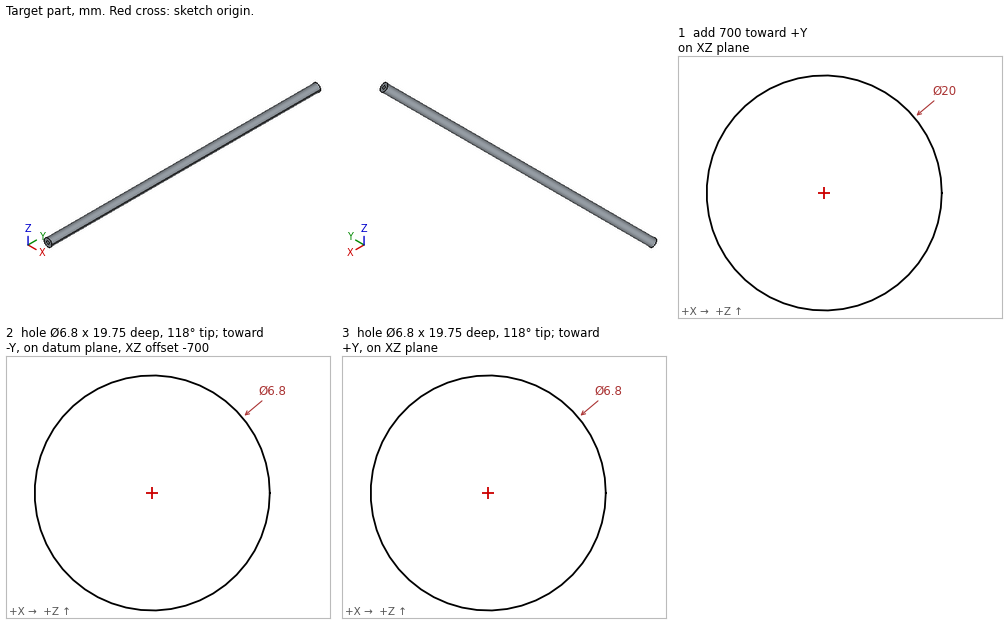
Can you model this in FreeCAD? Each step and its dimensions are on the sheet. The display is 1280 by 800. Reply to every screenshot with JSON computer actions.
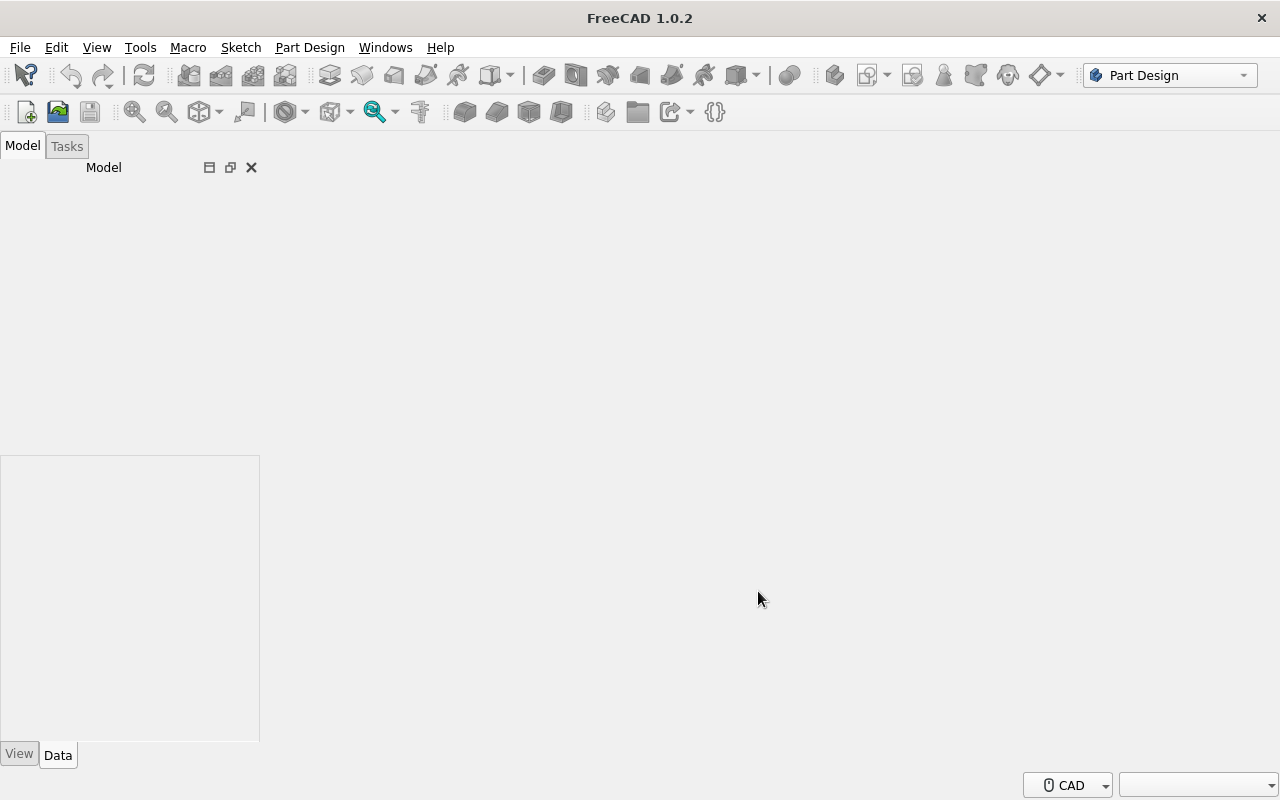
{"action": "left_click", "coordinate": [26, 112]}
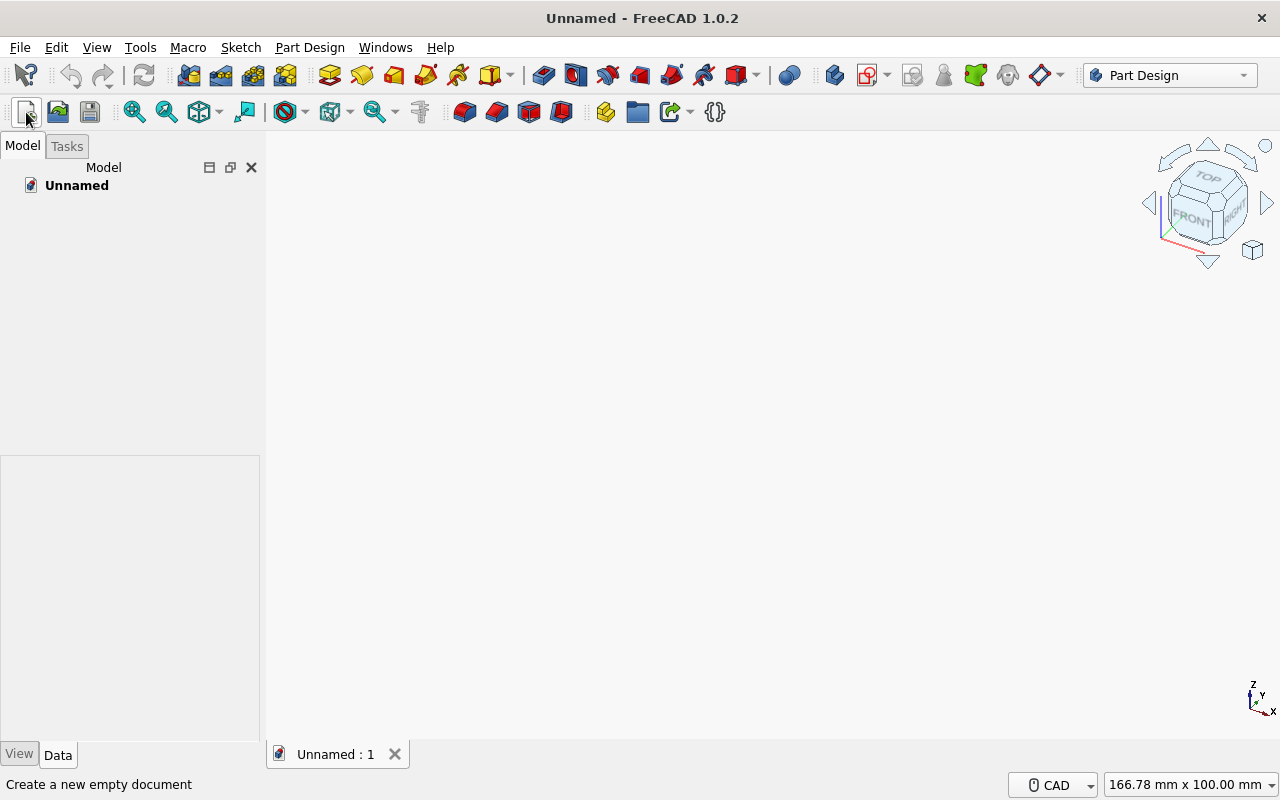
{"action": "left_click", "coordinate": [868, 76]}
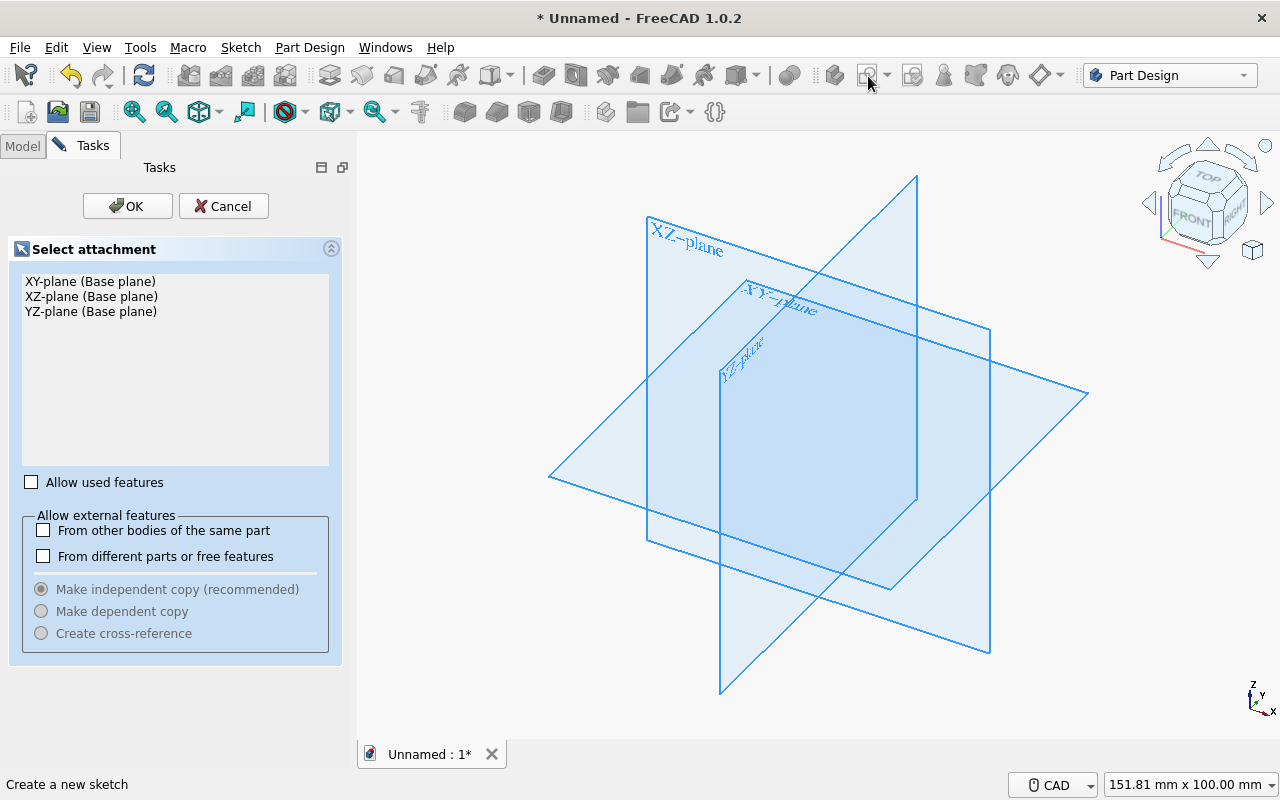
{"action": "left_click", "coordinate": [82, 296]}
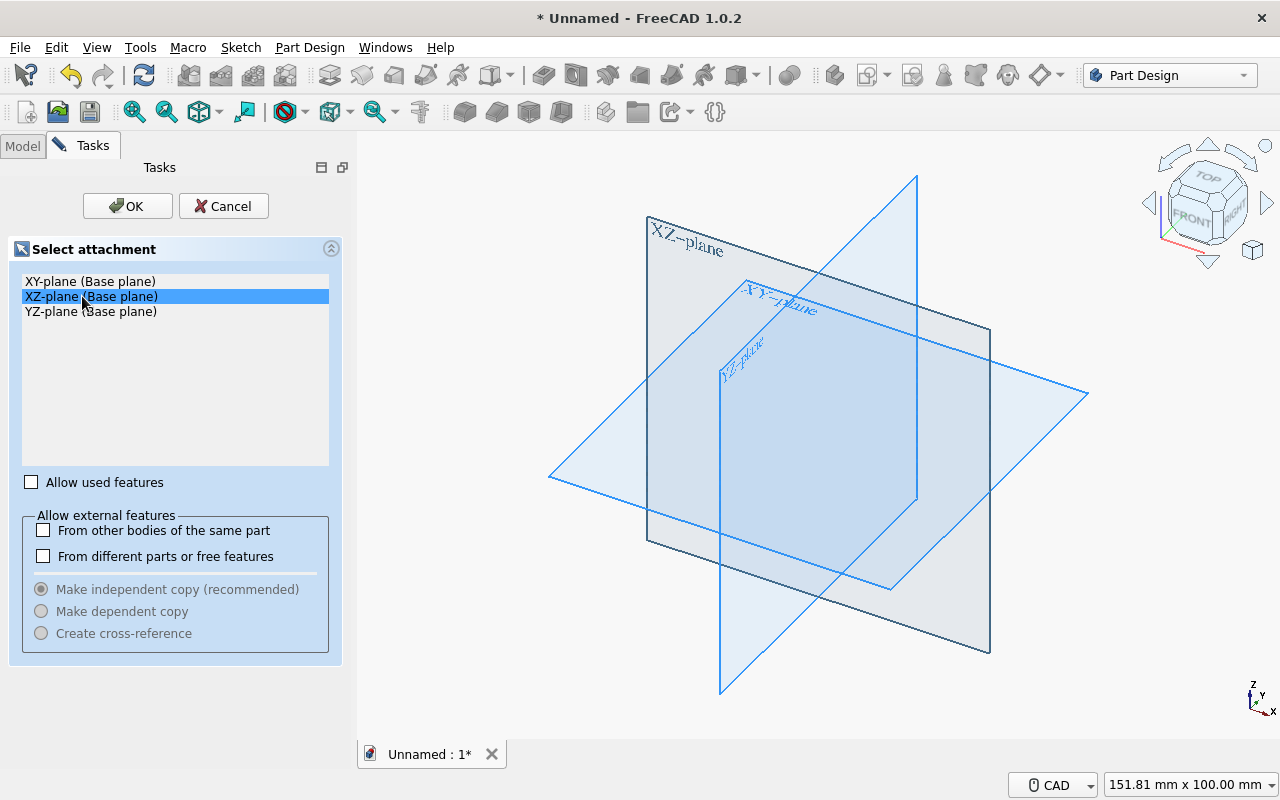
{"action": "left_click", "coordinate": [128, 206]}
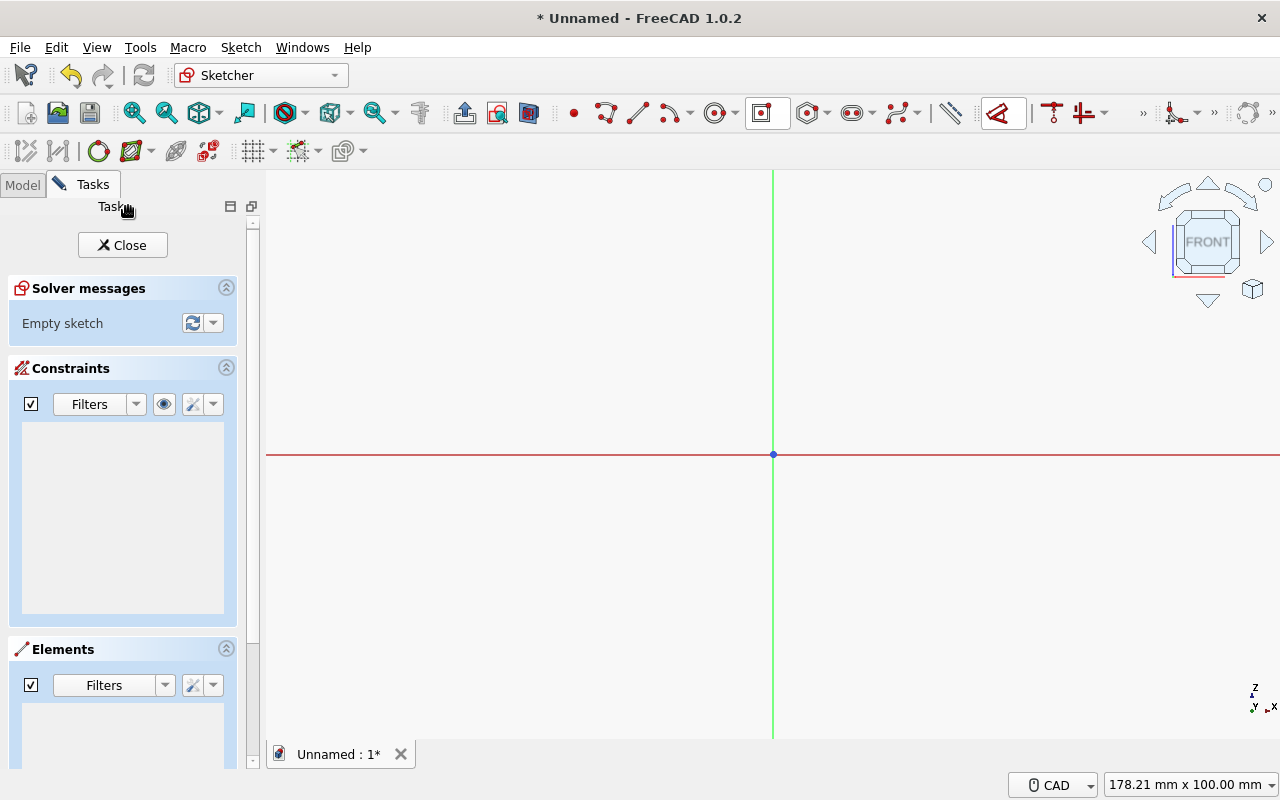
{"action": "scroll", "coordinate": [803, 455], "scroll_direction": "up", "scroll_amount": 6}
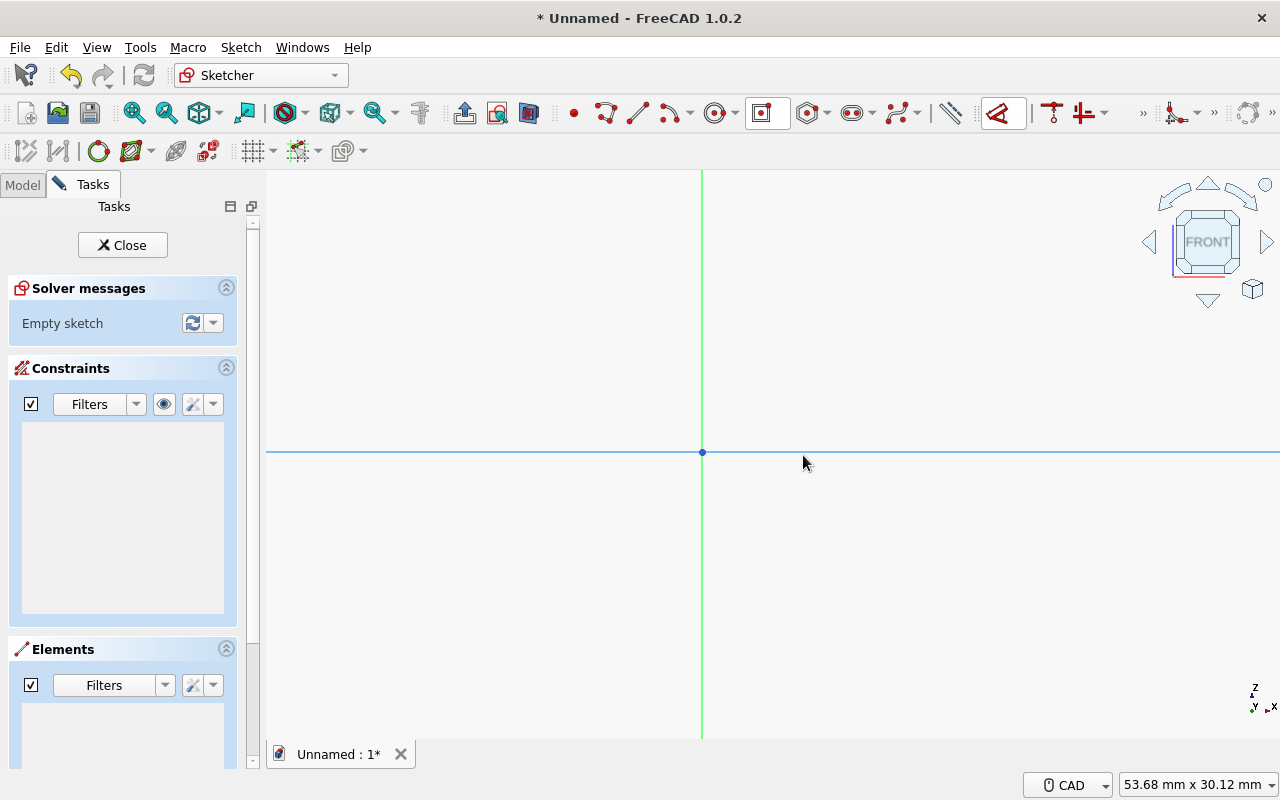
{"action": "left_click", "coordinate": [716, 114]}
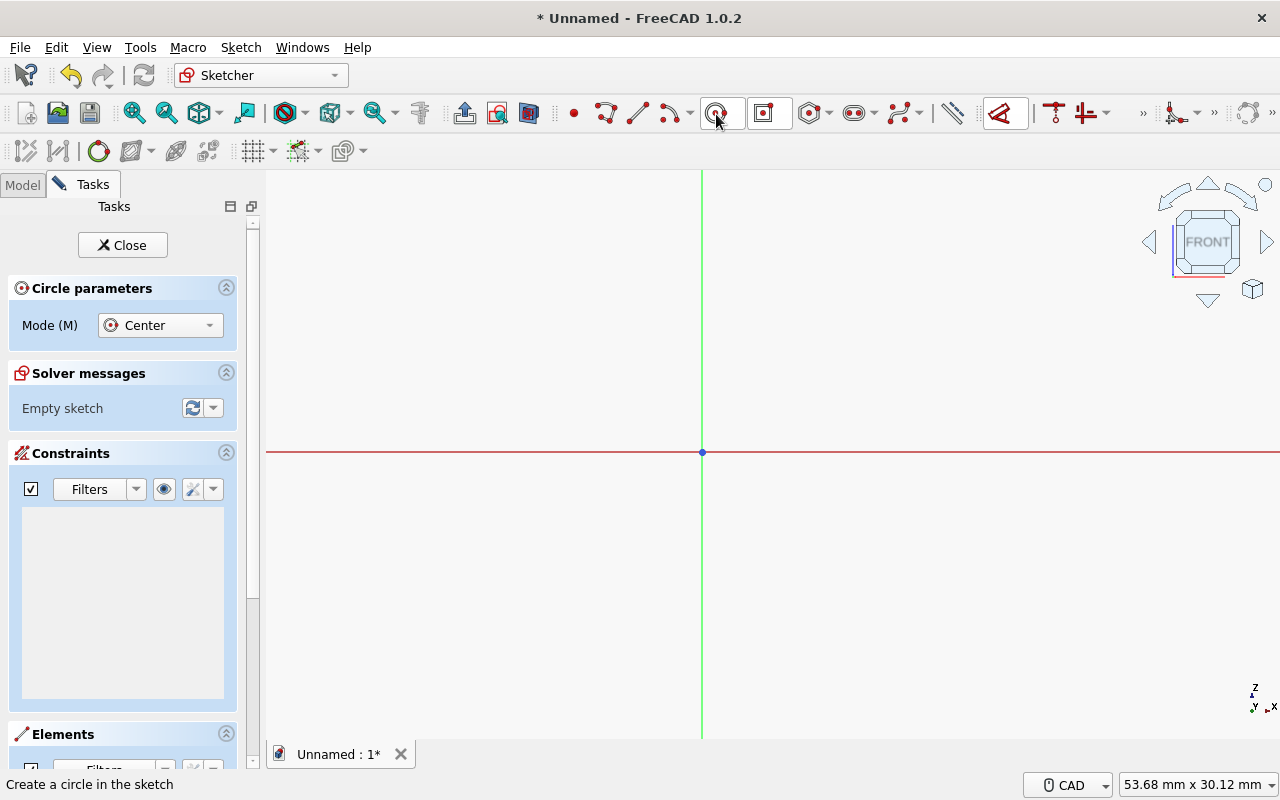
{"action": "left_click", "coordinate": [702, 452]}
{"action": "mouse_move", "coordinate": [836, 319]}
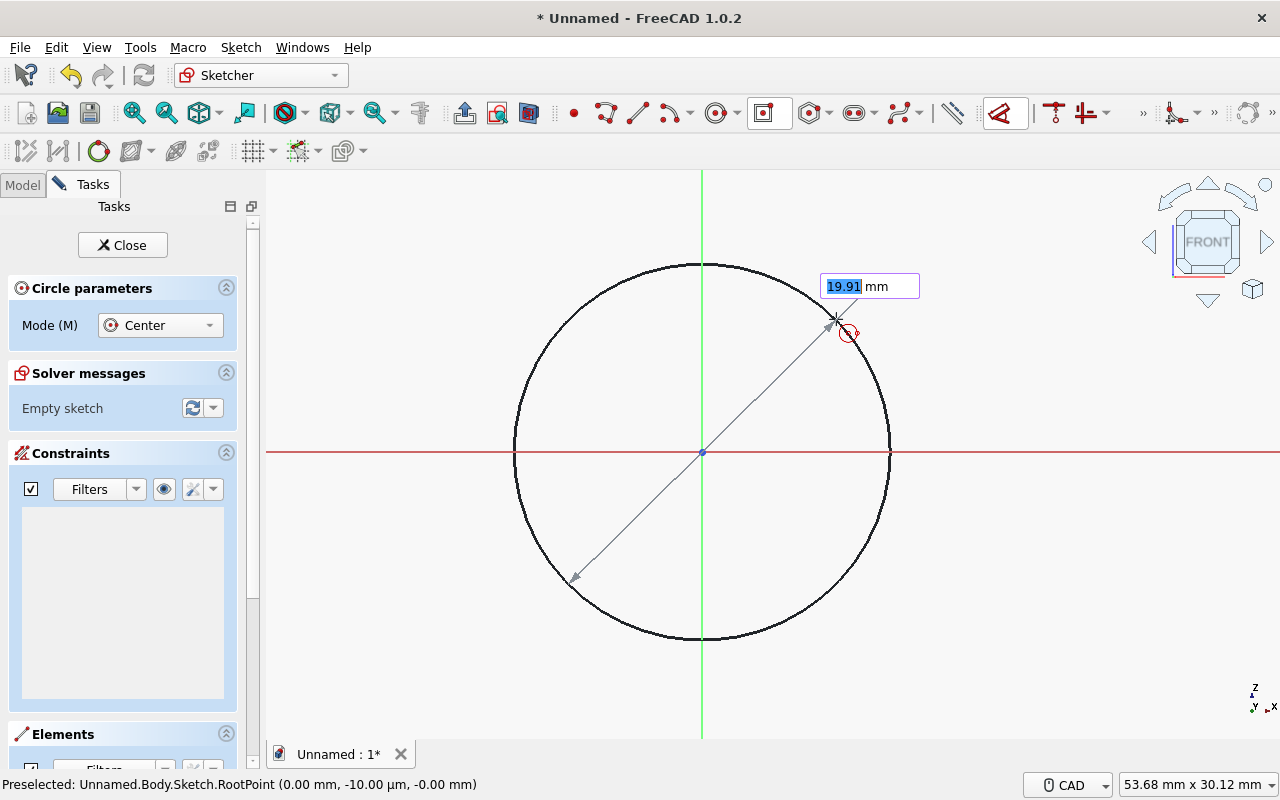
{"action": "type", "text": "20"}
{"action": "key", "text": "Return"}
{"action": "key", "text": "Escape"}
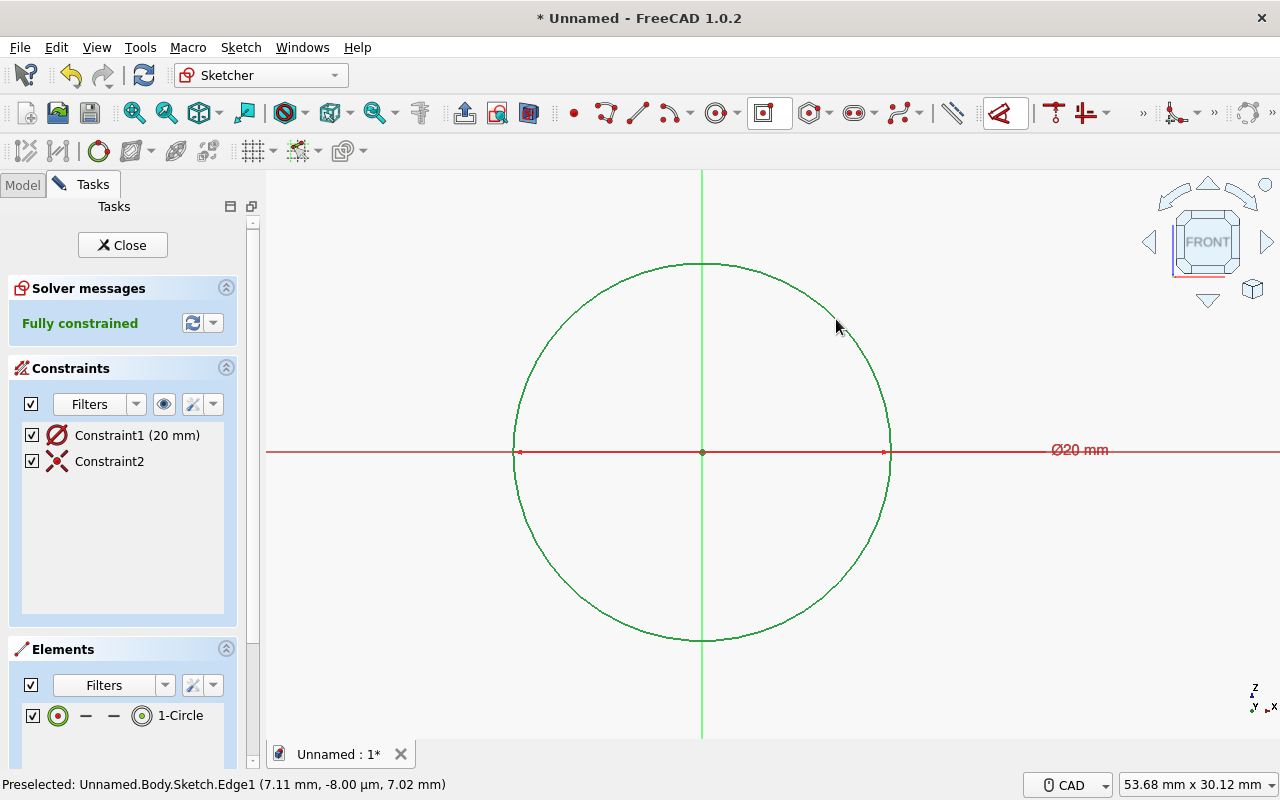
{"action": "left_click", "coordinate": [123, 245]}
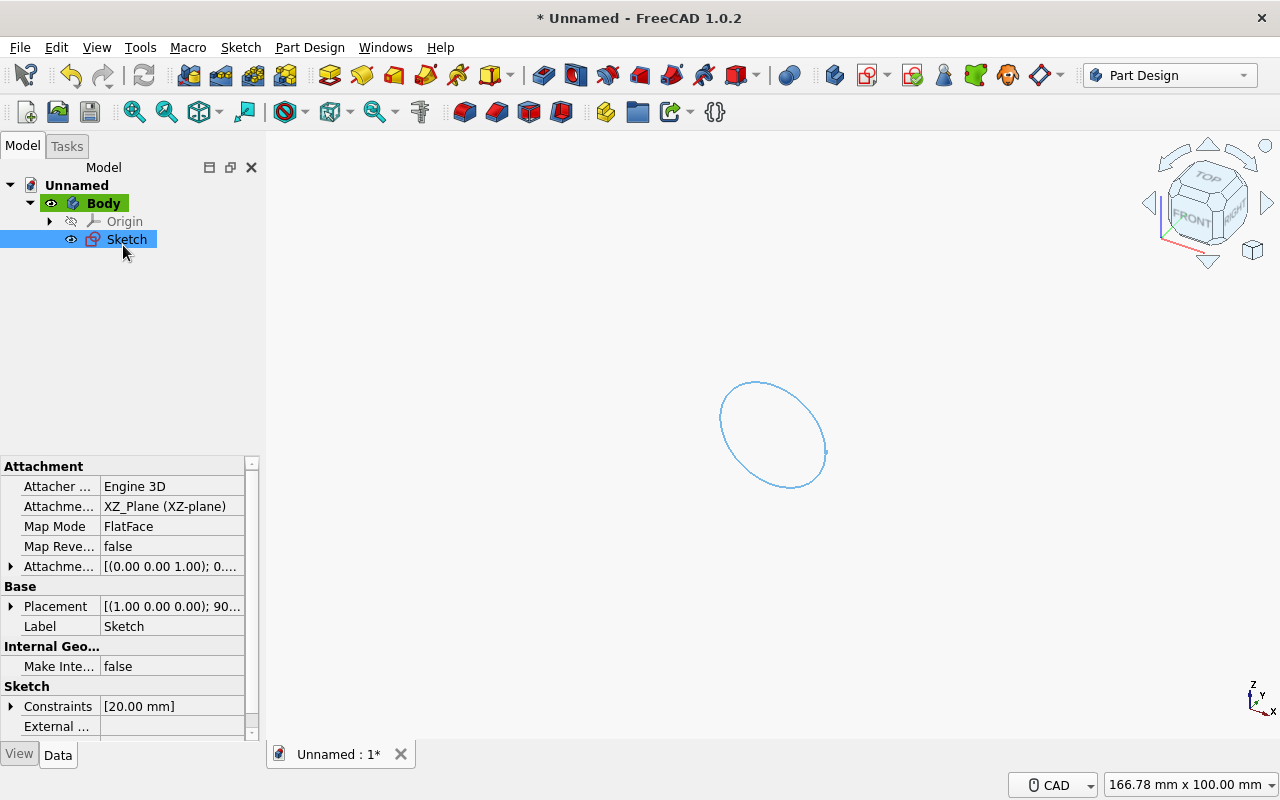
{"action": "left_click", "coordinate": [330, 76]}